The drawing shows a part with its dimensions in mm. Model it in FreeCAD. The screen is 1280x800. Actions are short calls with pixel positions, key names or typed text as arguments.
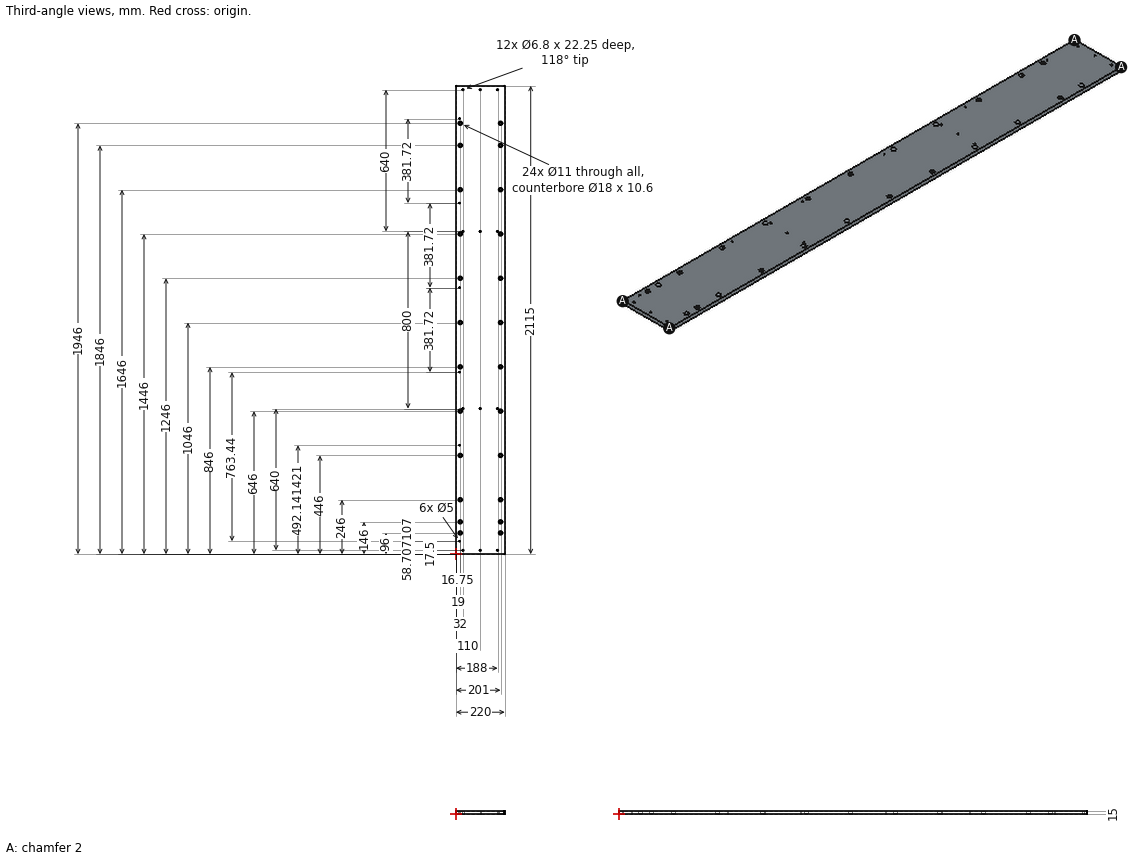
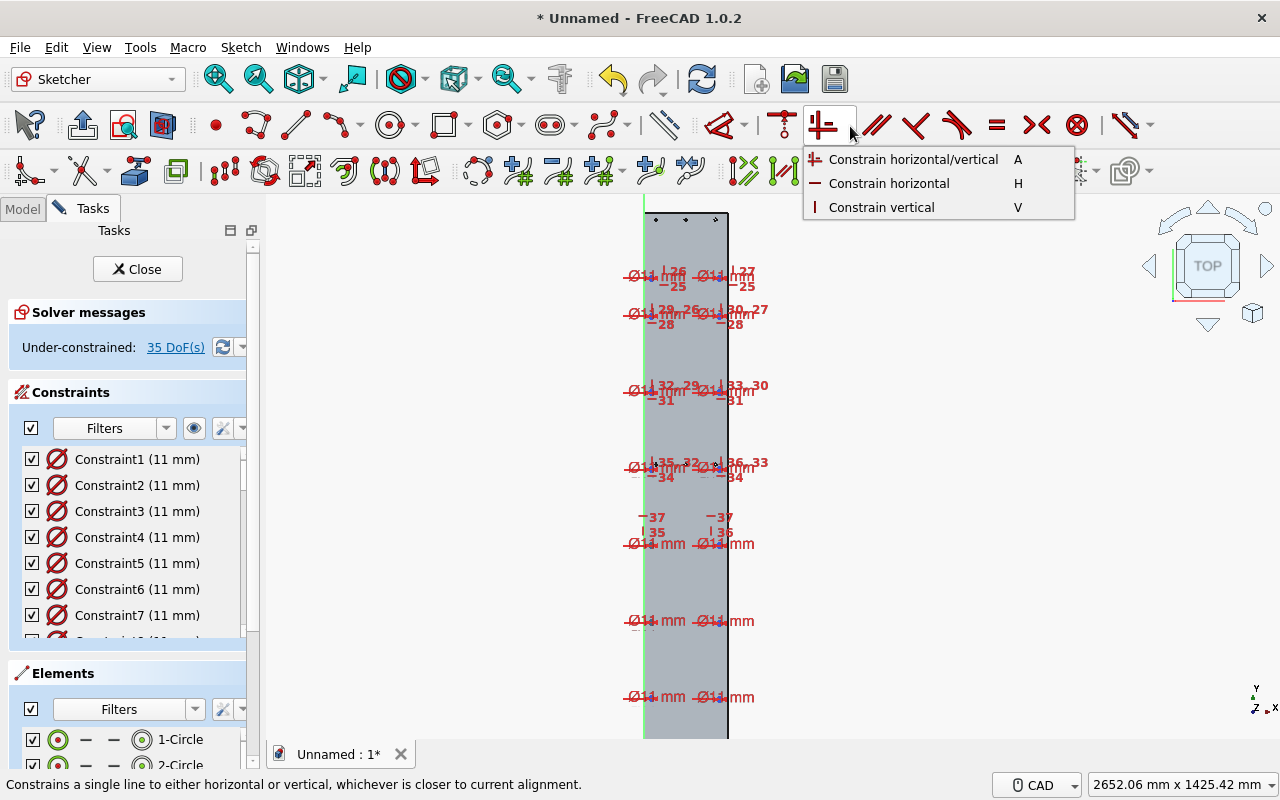
click(939, 207)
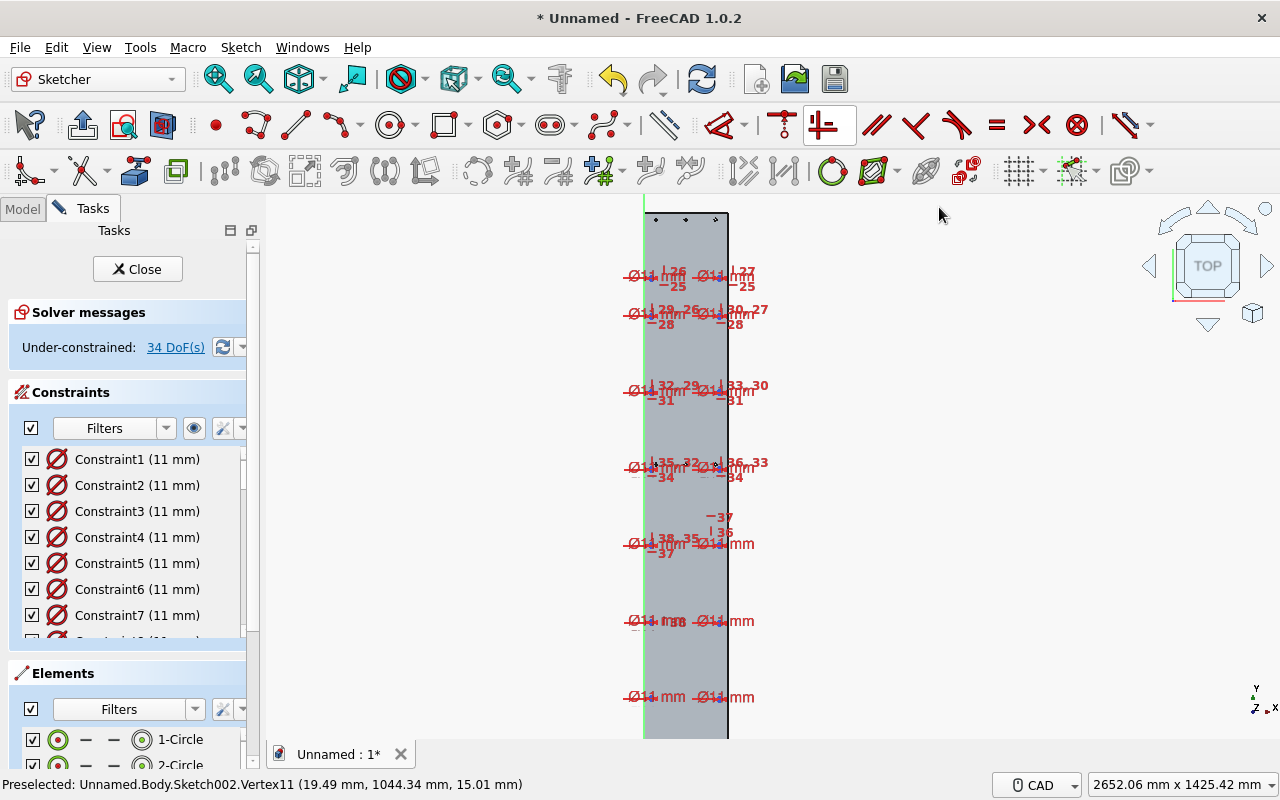
click(720, 546)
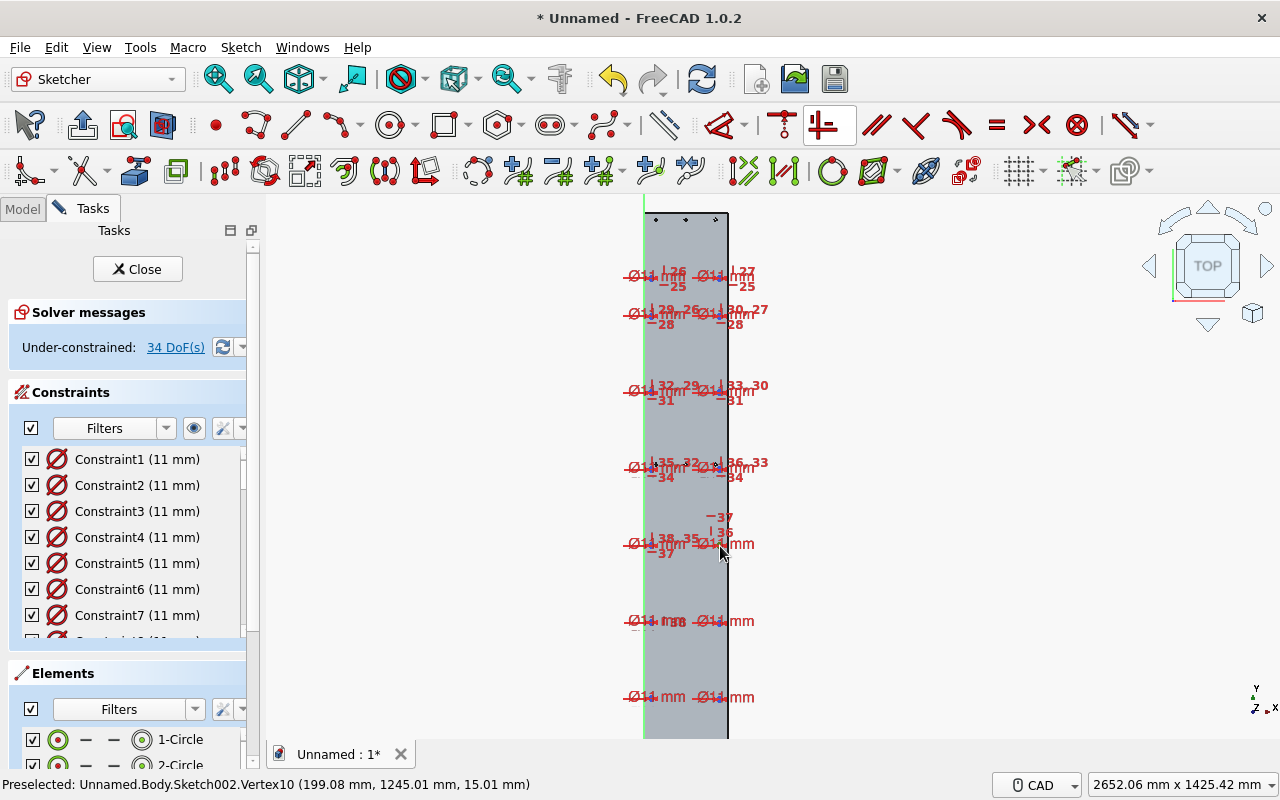
click(720, 623)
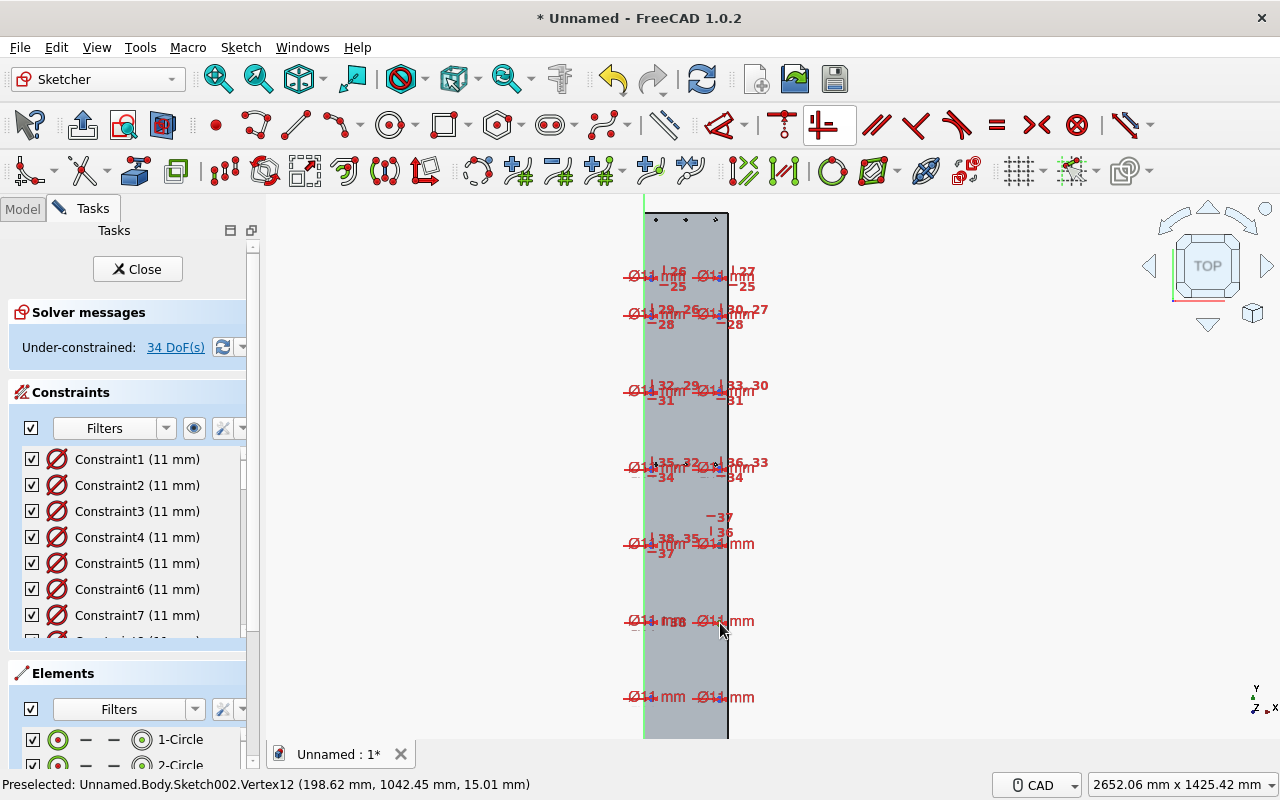
click(850, 126)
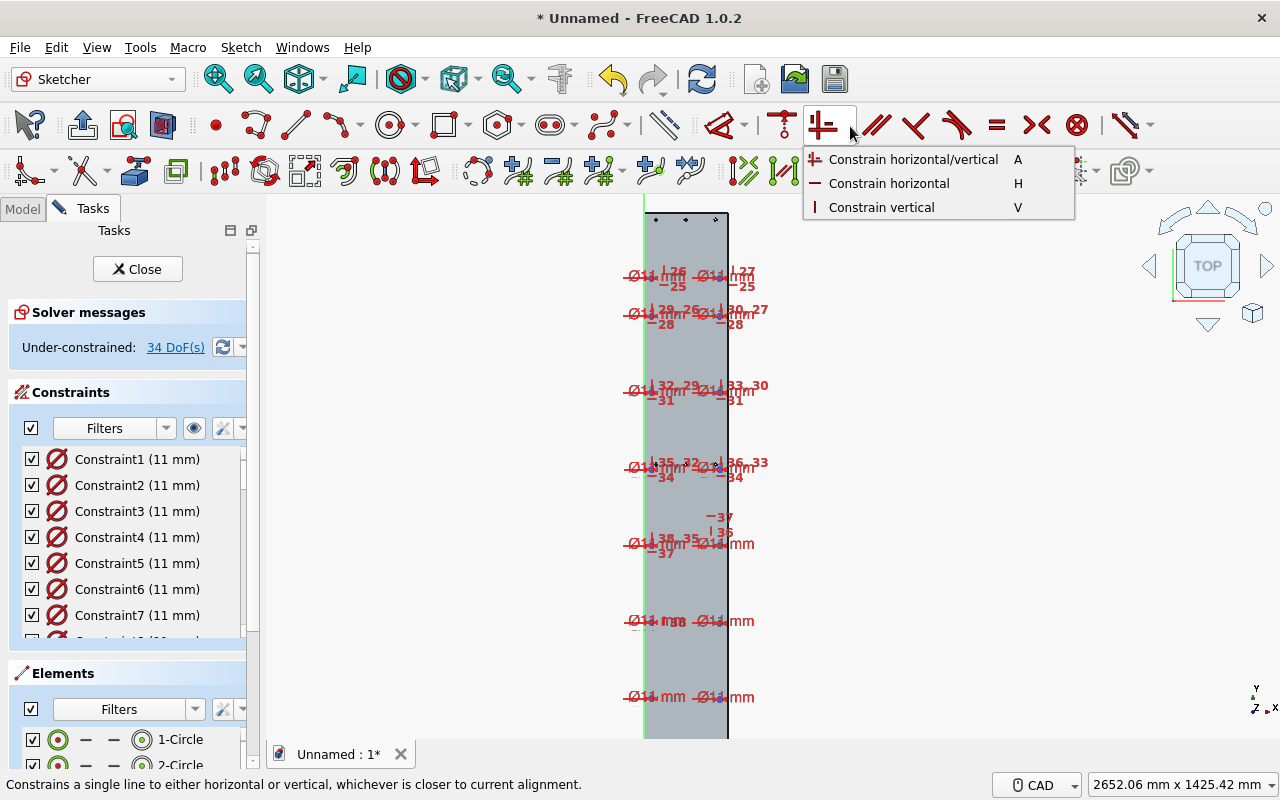
click(939, 207)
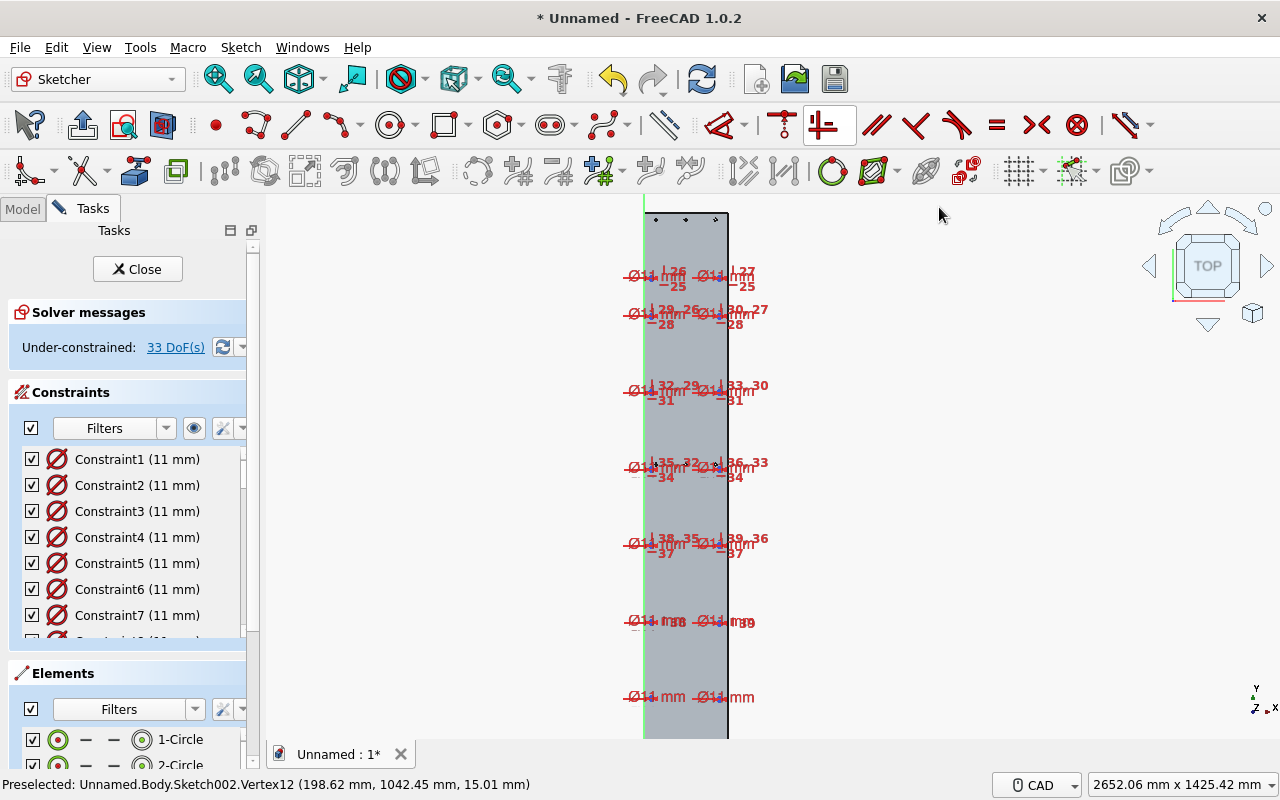
click(651, 623)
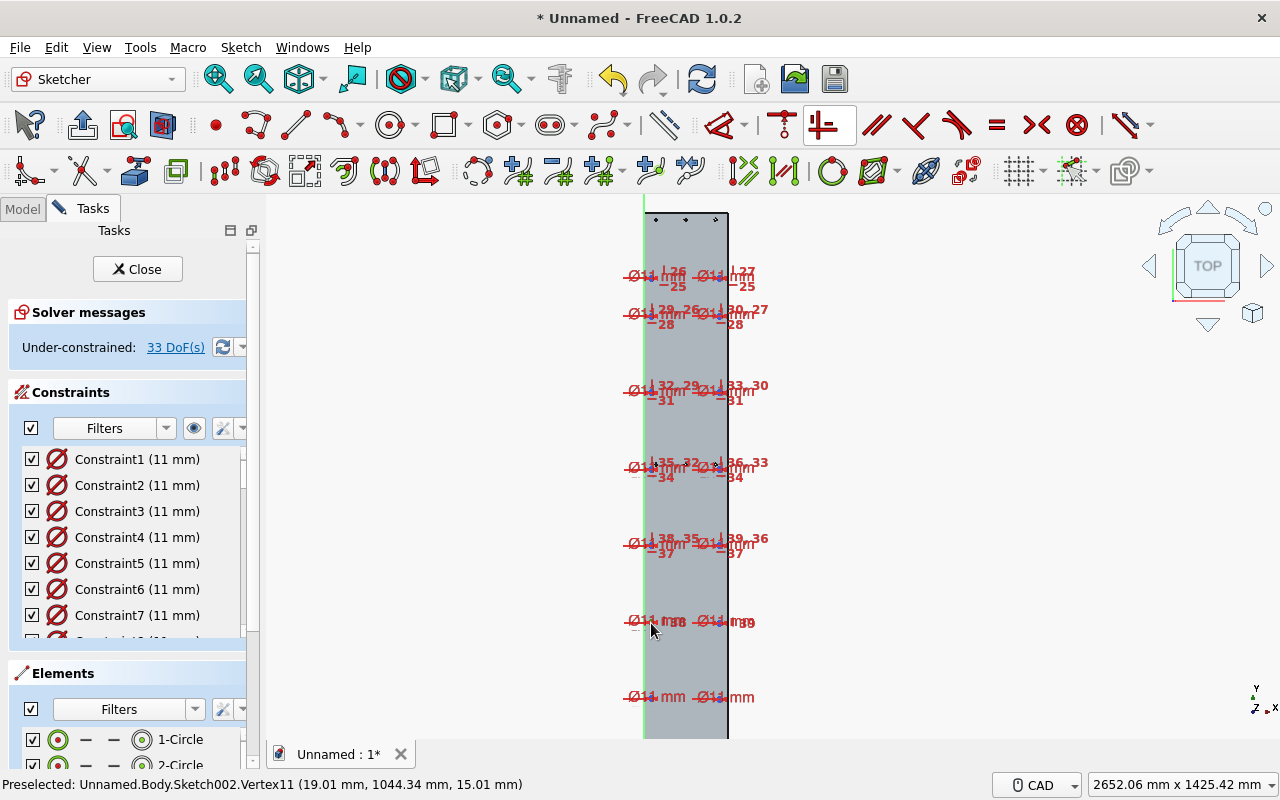
click(720, 623)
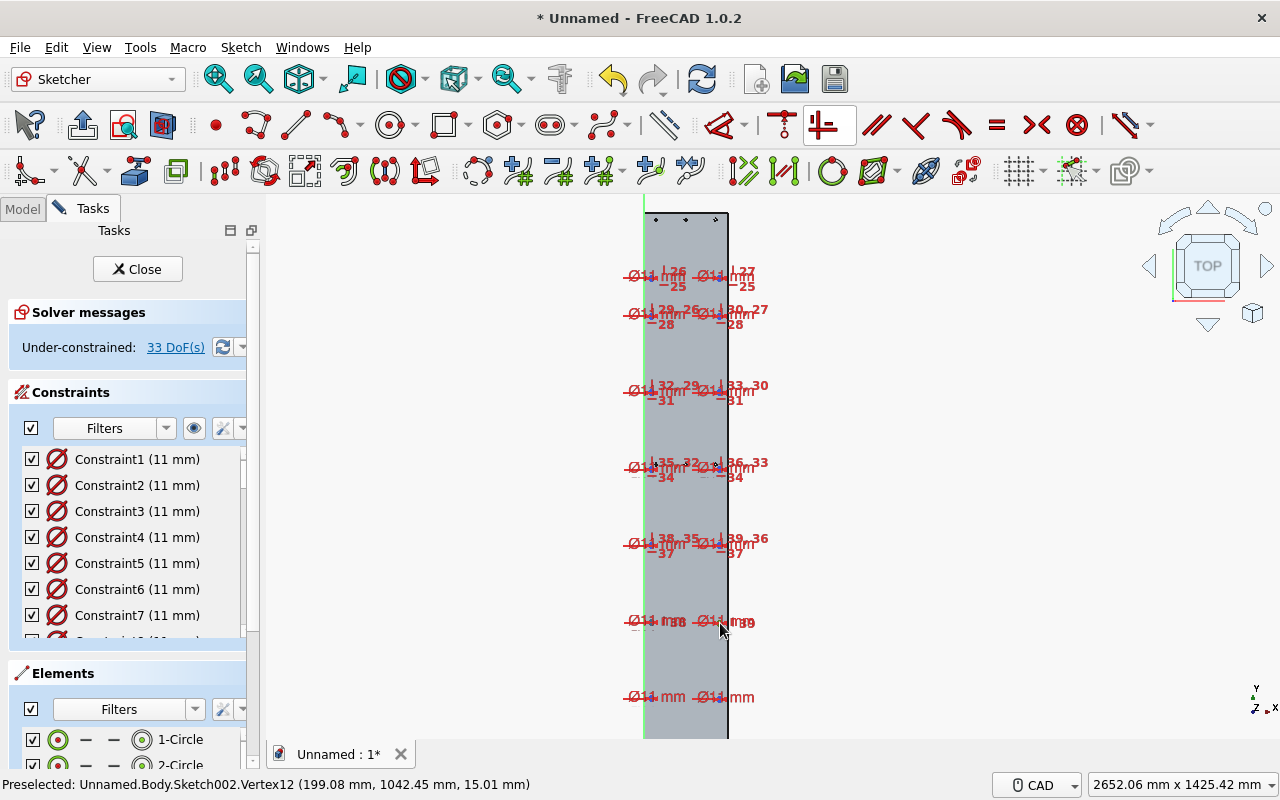
click(850, 126)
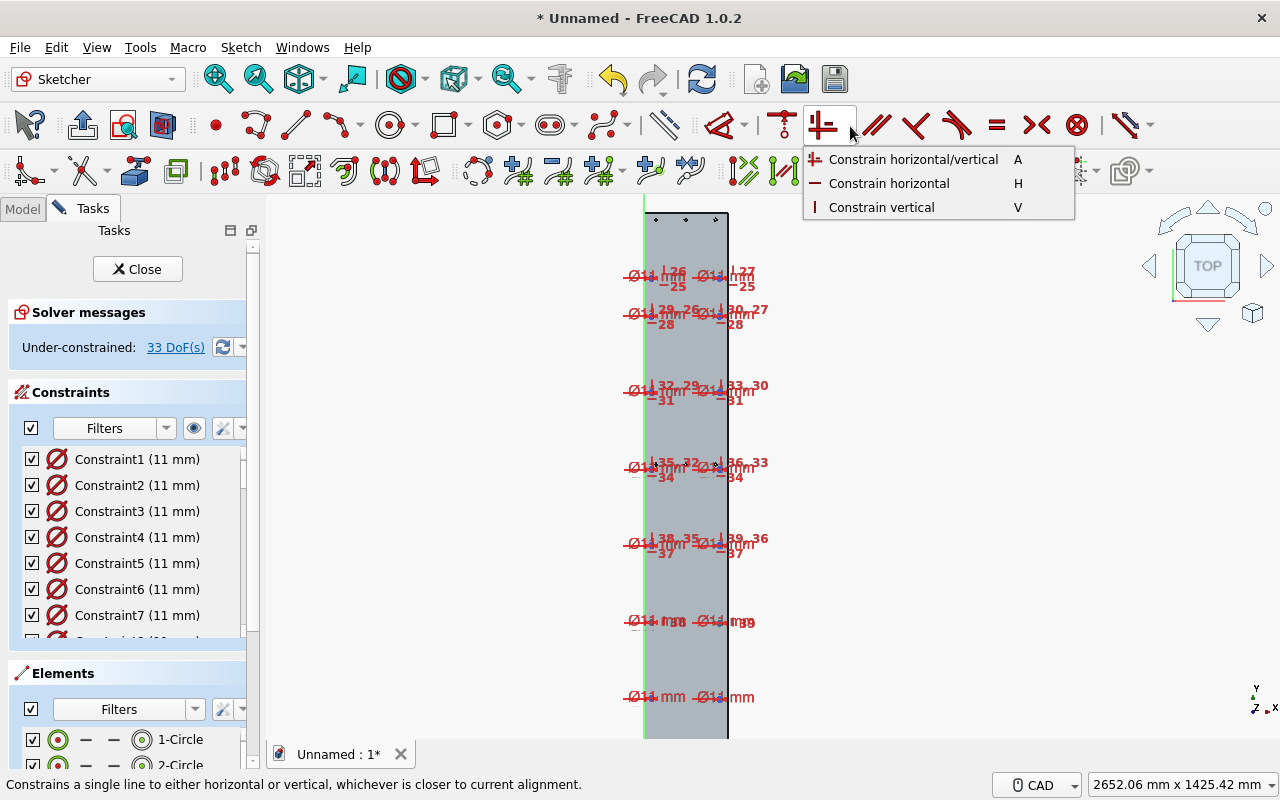
click(939, 183)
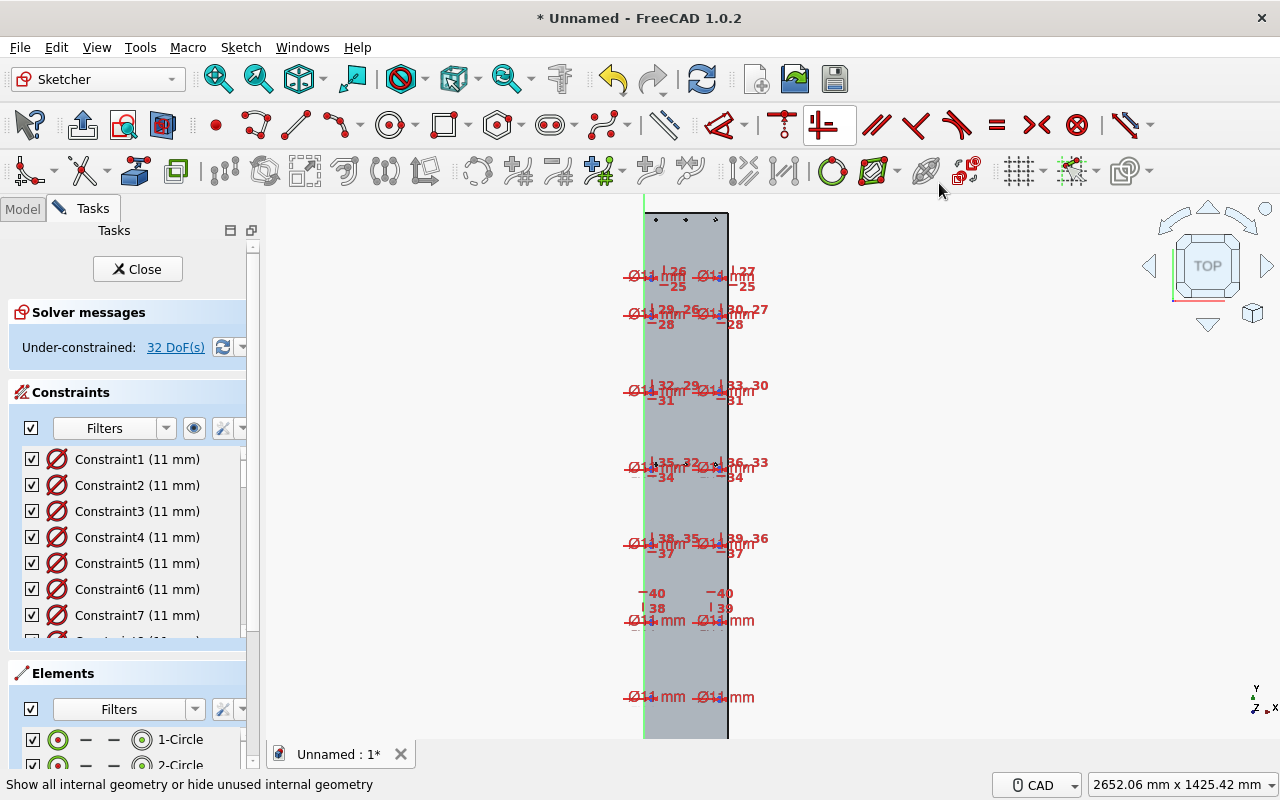
click(651, 623)